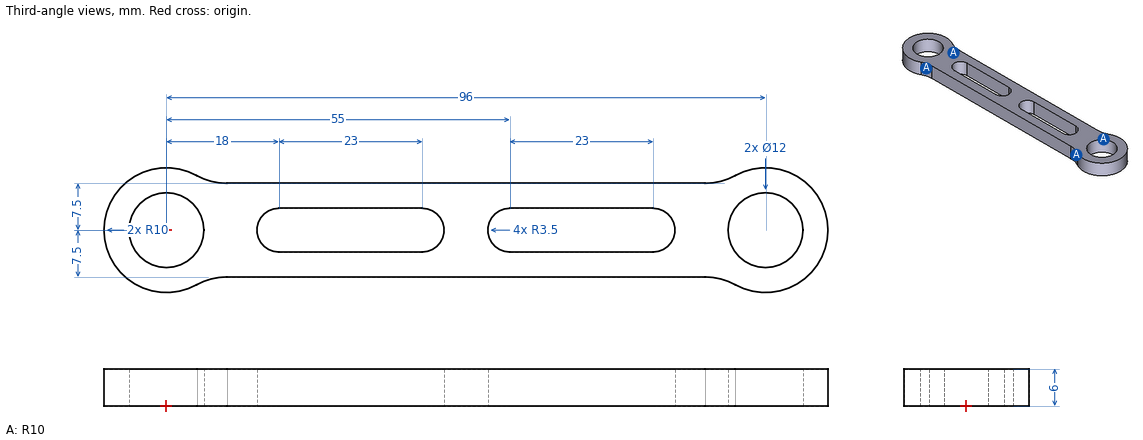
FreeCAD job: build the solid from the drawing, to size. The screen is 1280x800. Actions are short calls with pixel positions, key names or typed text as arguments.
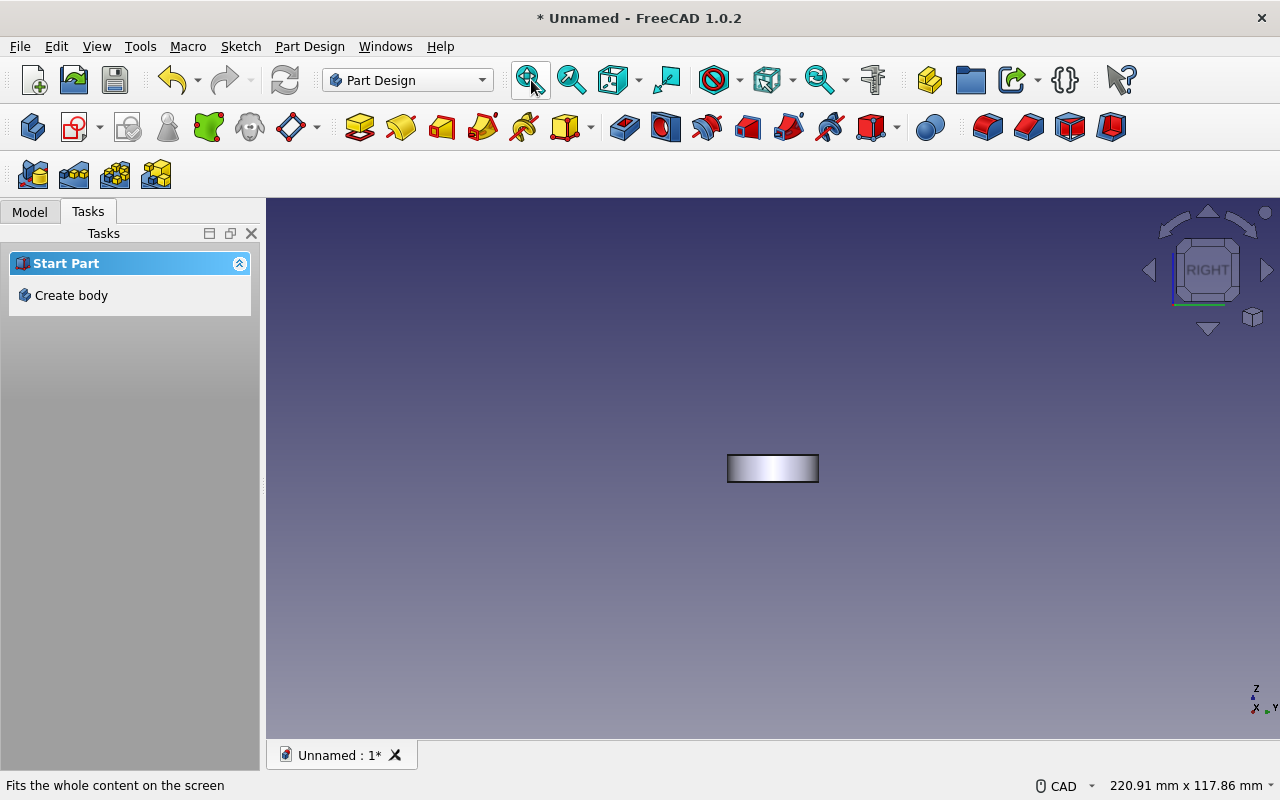
click(531, 80)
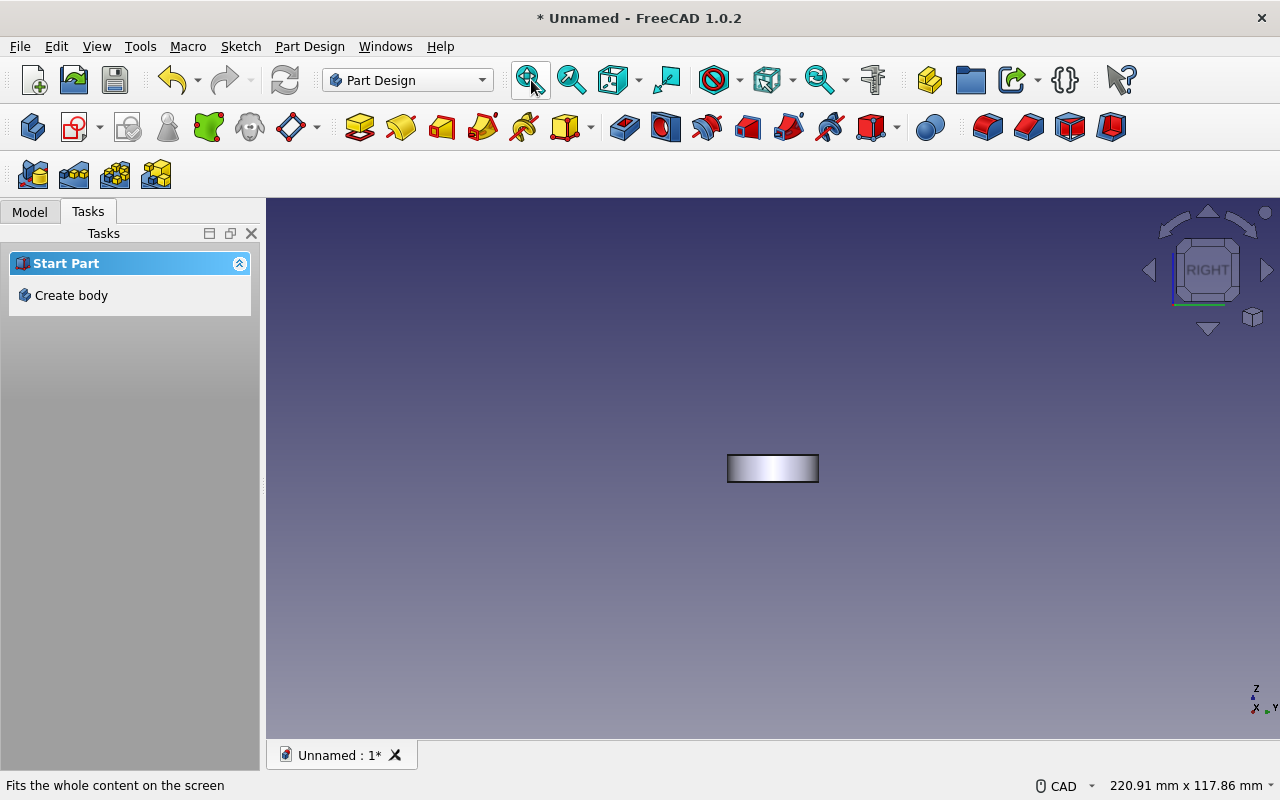
key(5)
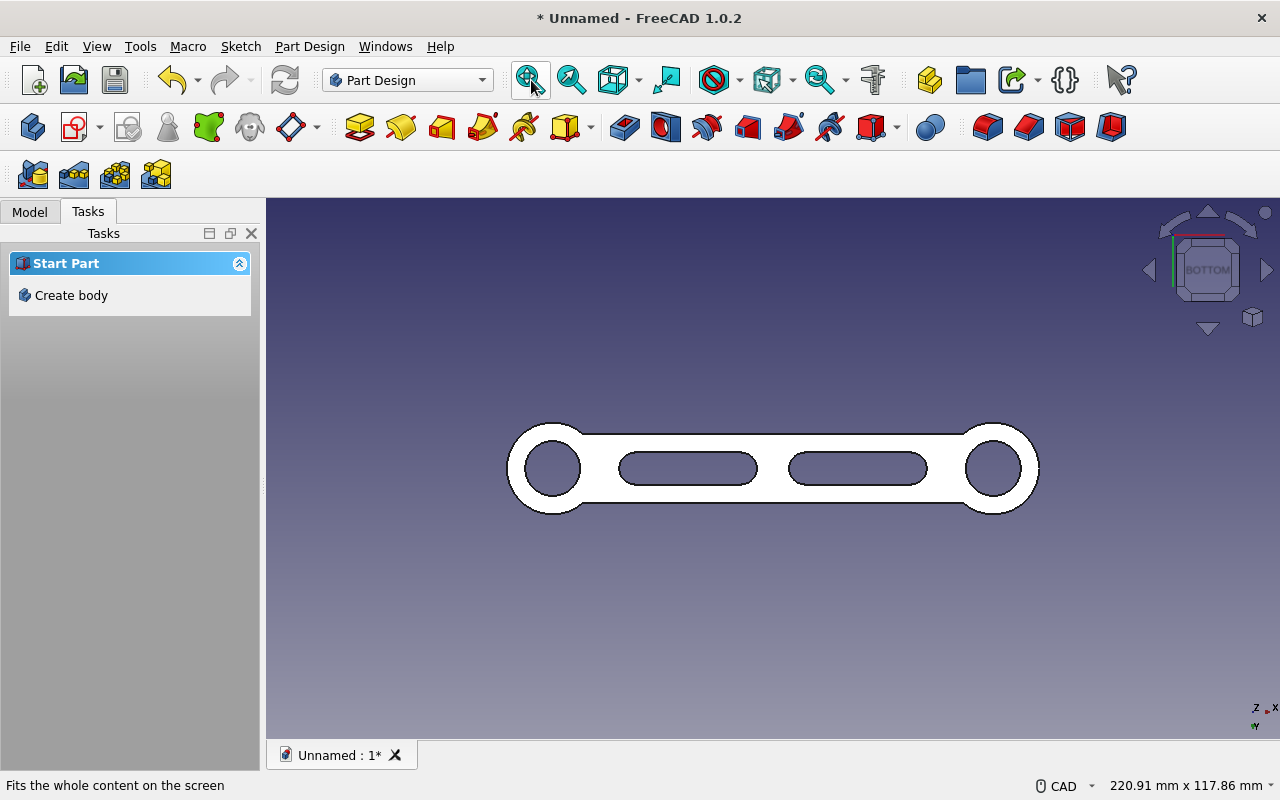
key(4)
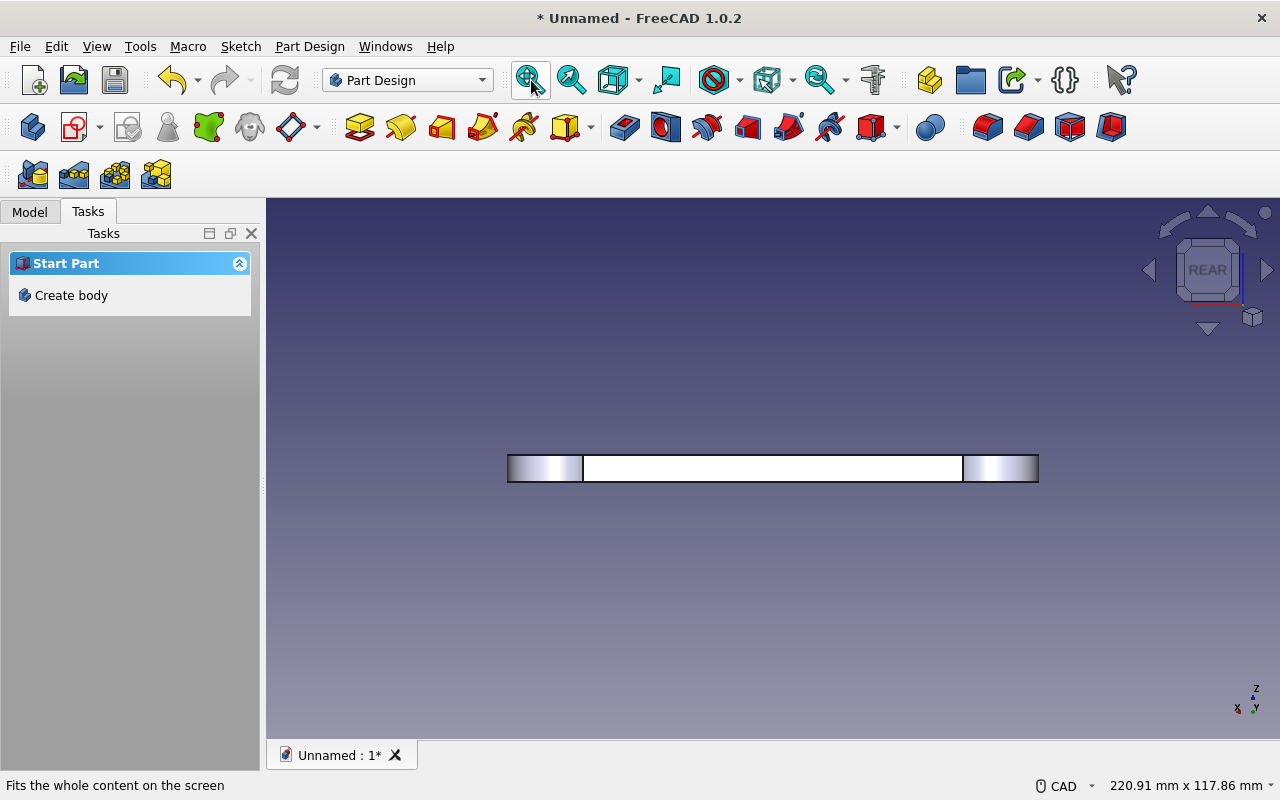
key(6)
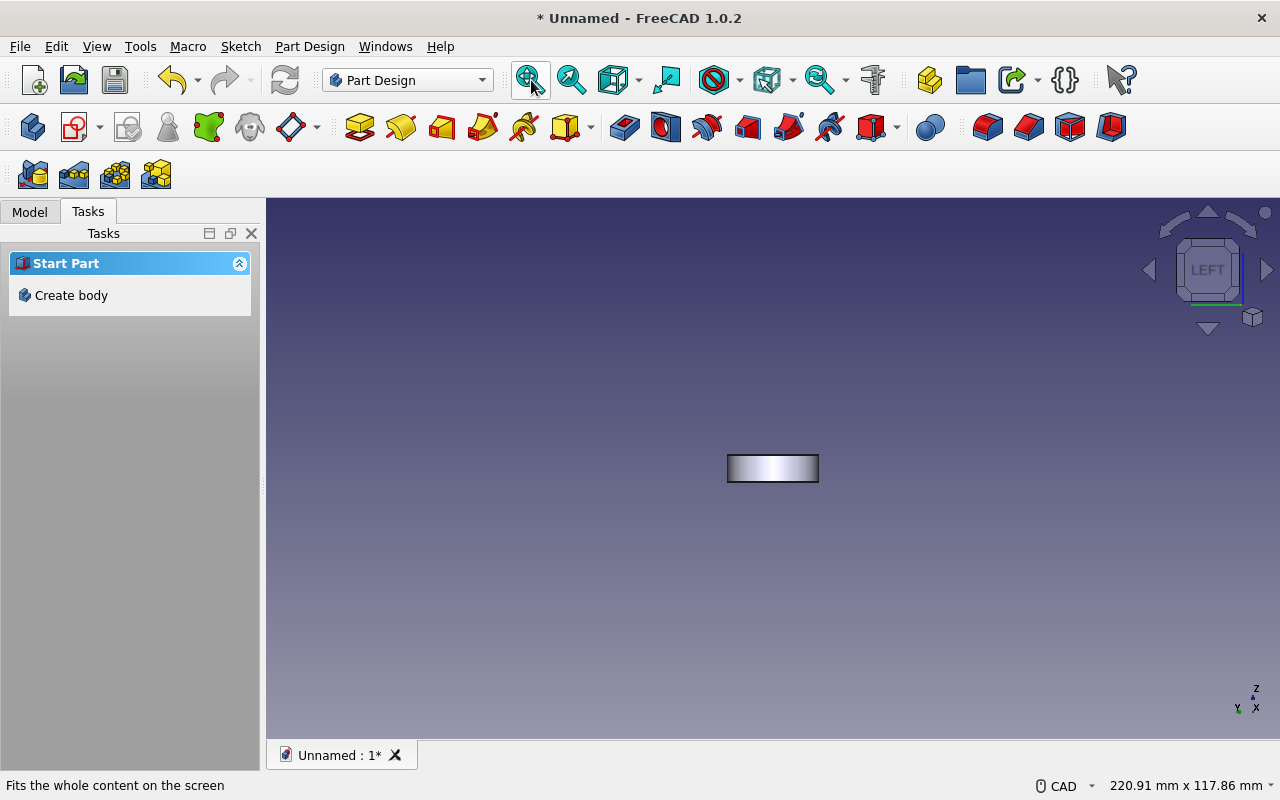
key(v)
key(f)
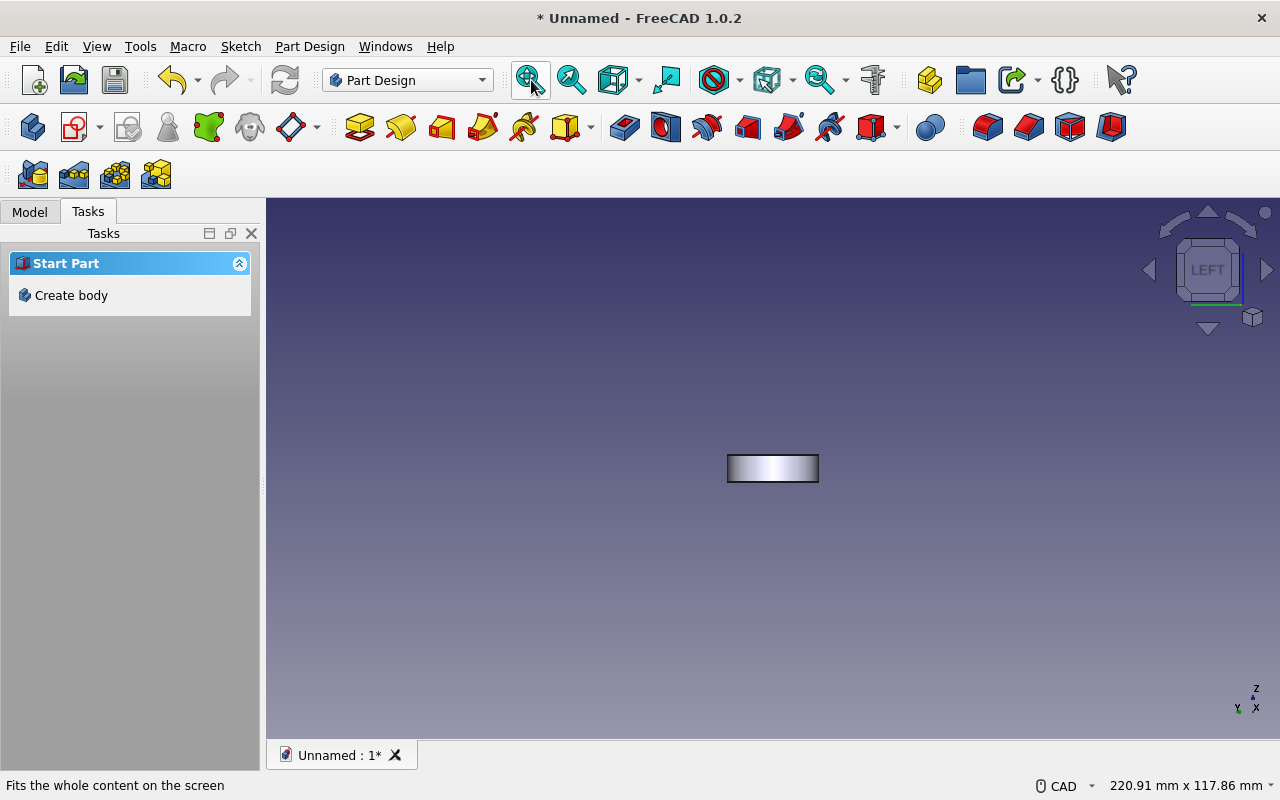
key(v)
key(3)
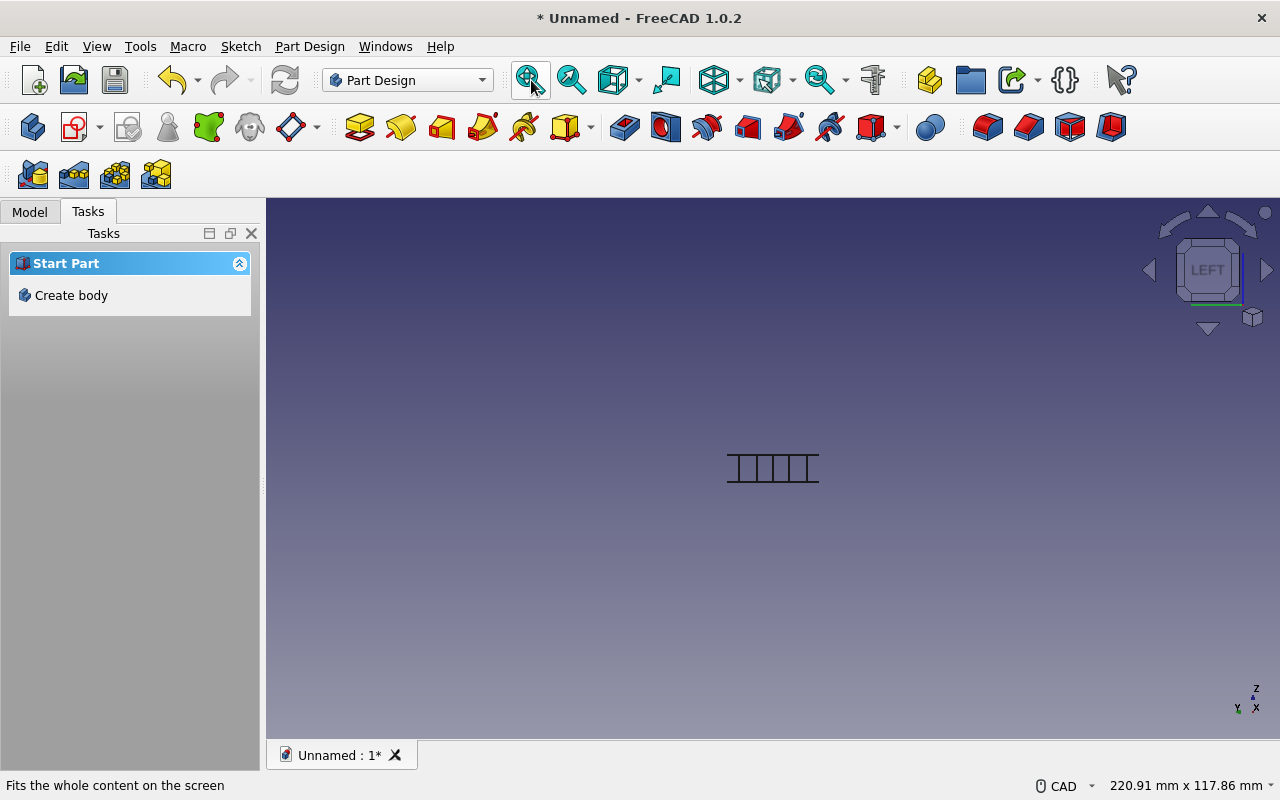
key(0)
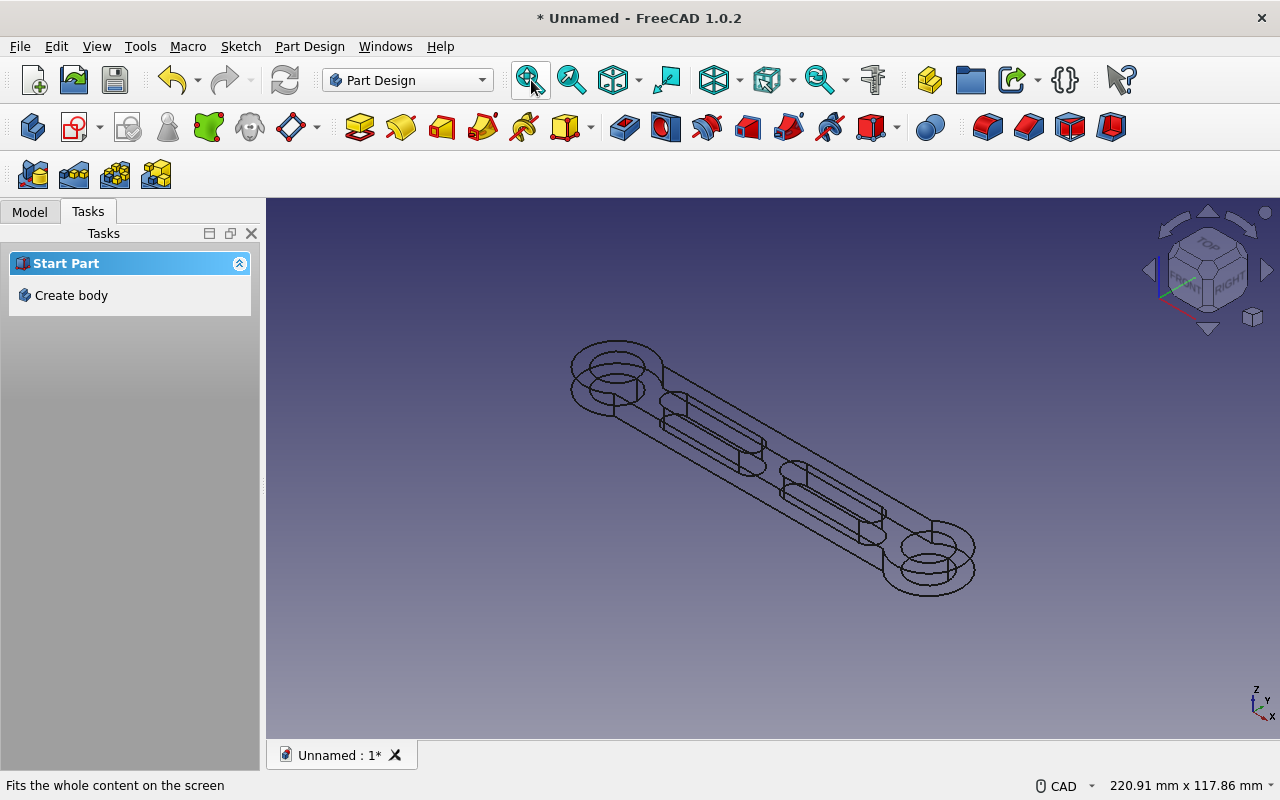
click(663, 376)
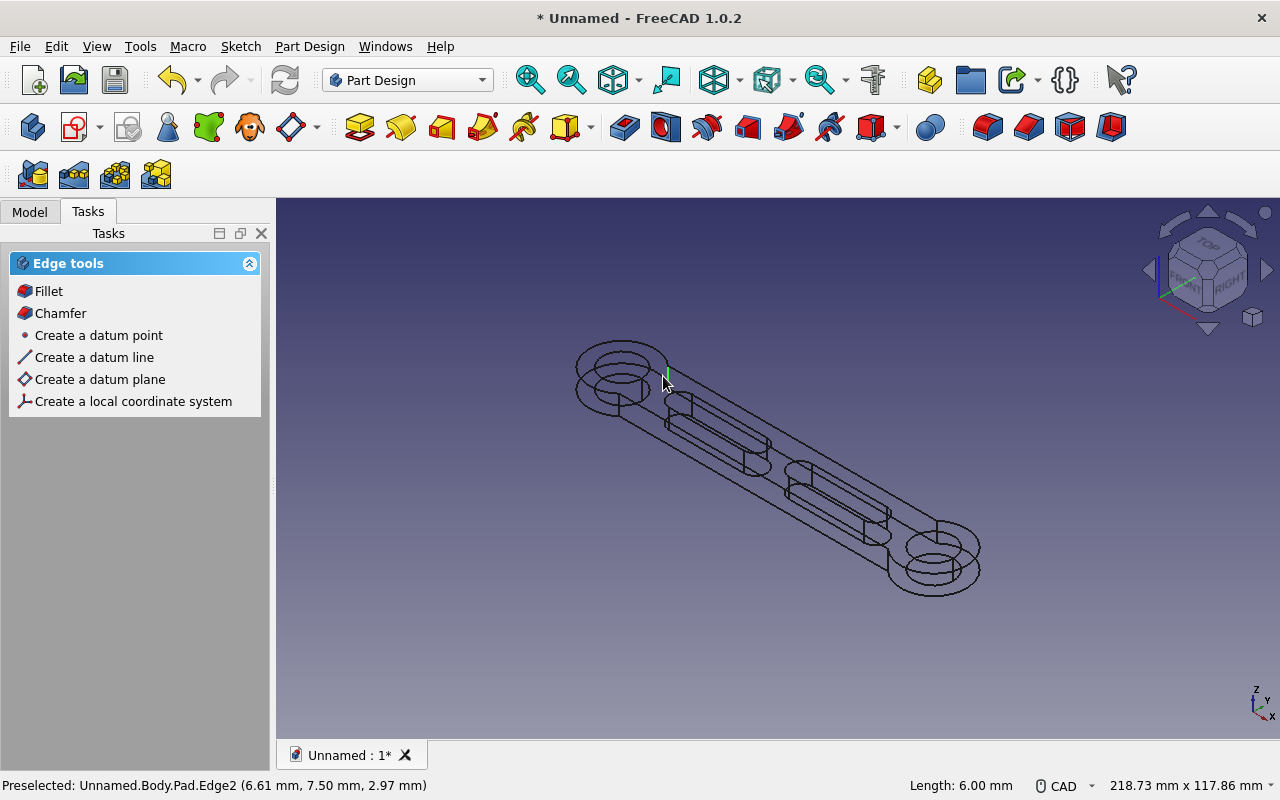
click(937, 538, ctrl)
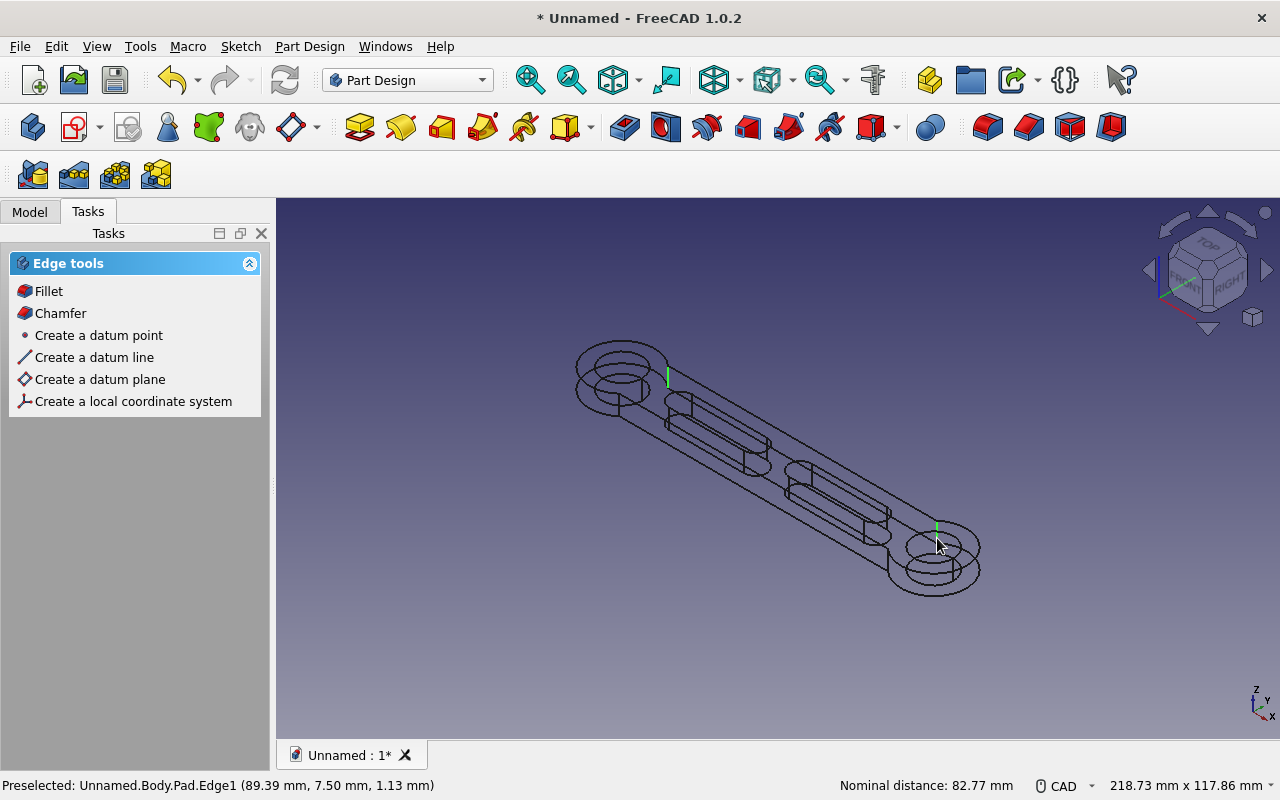
click(888, 564, ctrl)